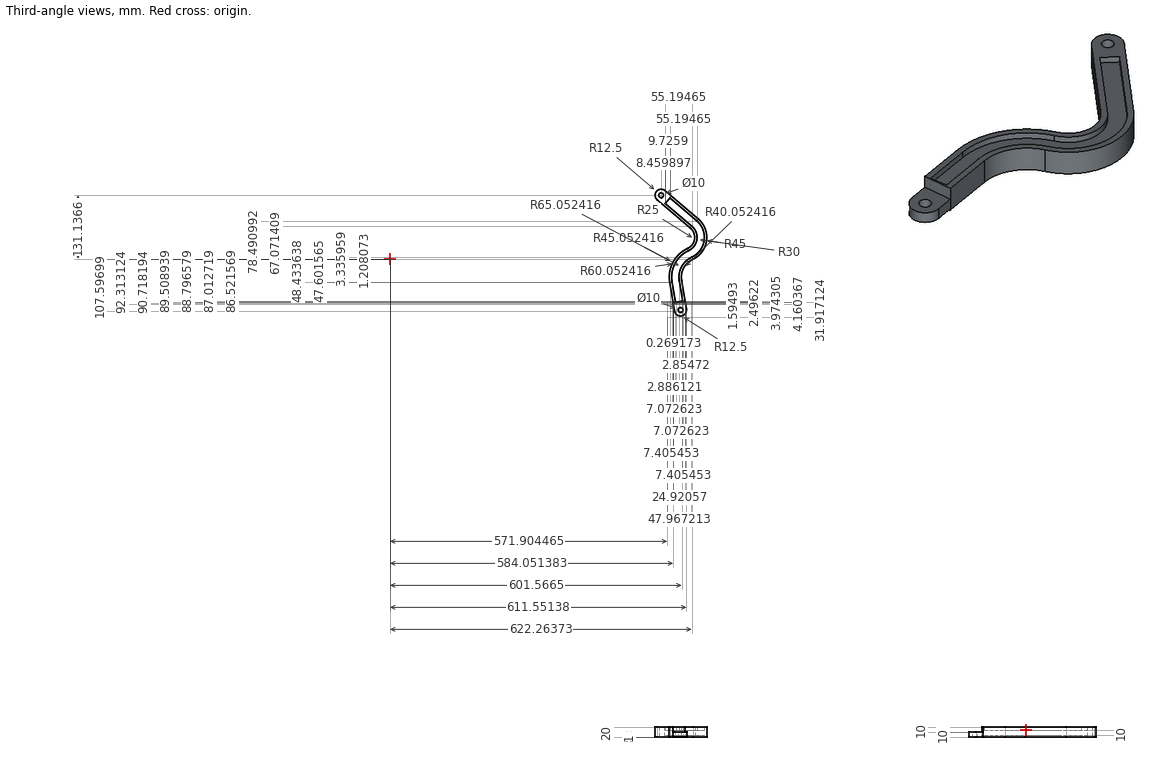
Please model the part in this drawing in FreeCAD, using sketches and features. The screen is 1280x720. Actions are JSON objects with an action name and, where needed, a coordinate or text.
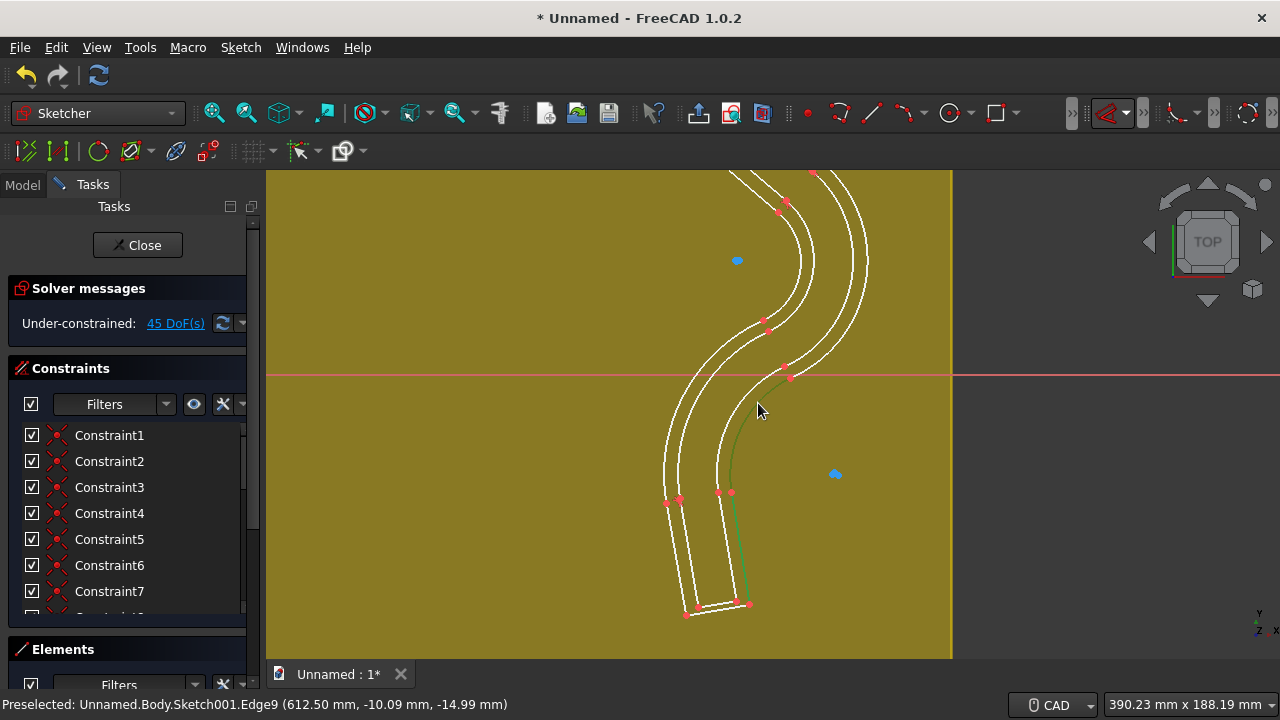
{"action": "key", "text": "t"}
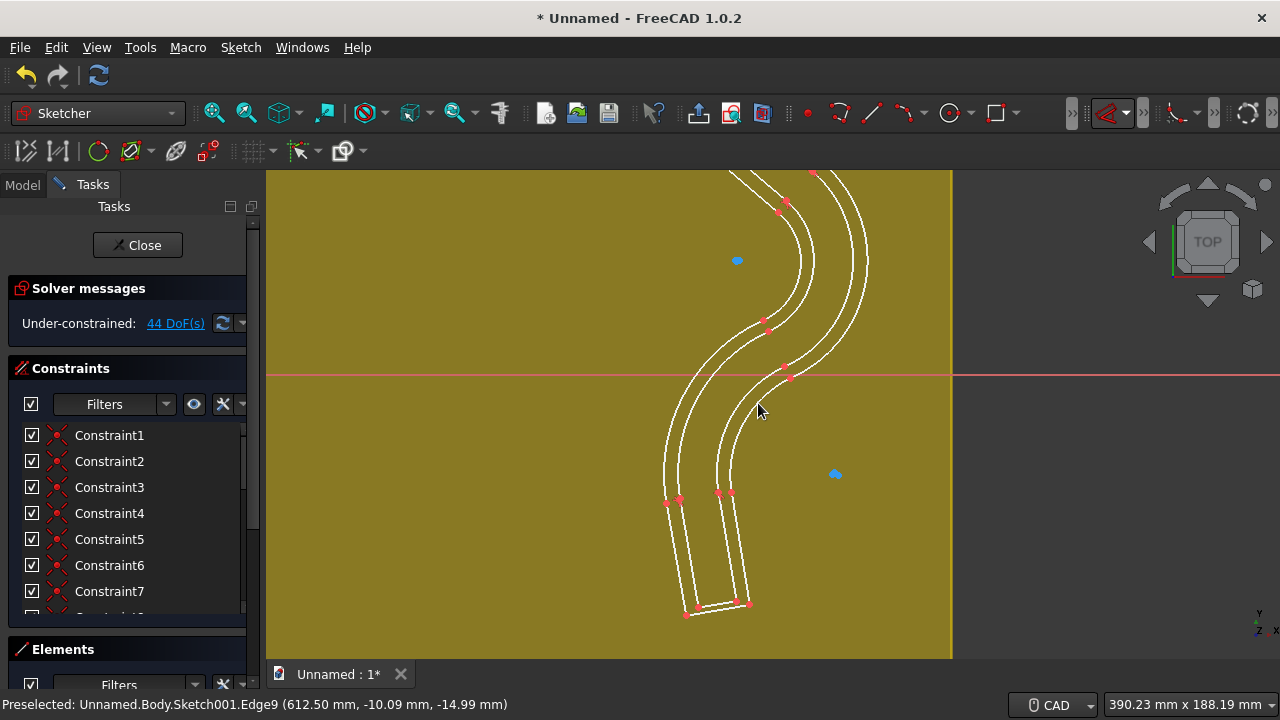
{"action": "left_click", "coordinate": [792, 294]}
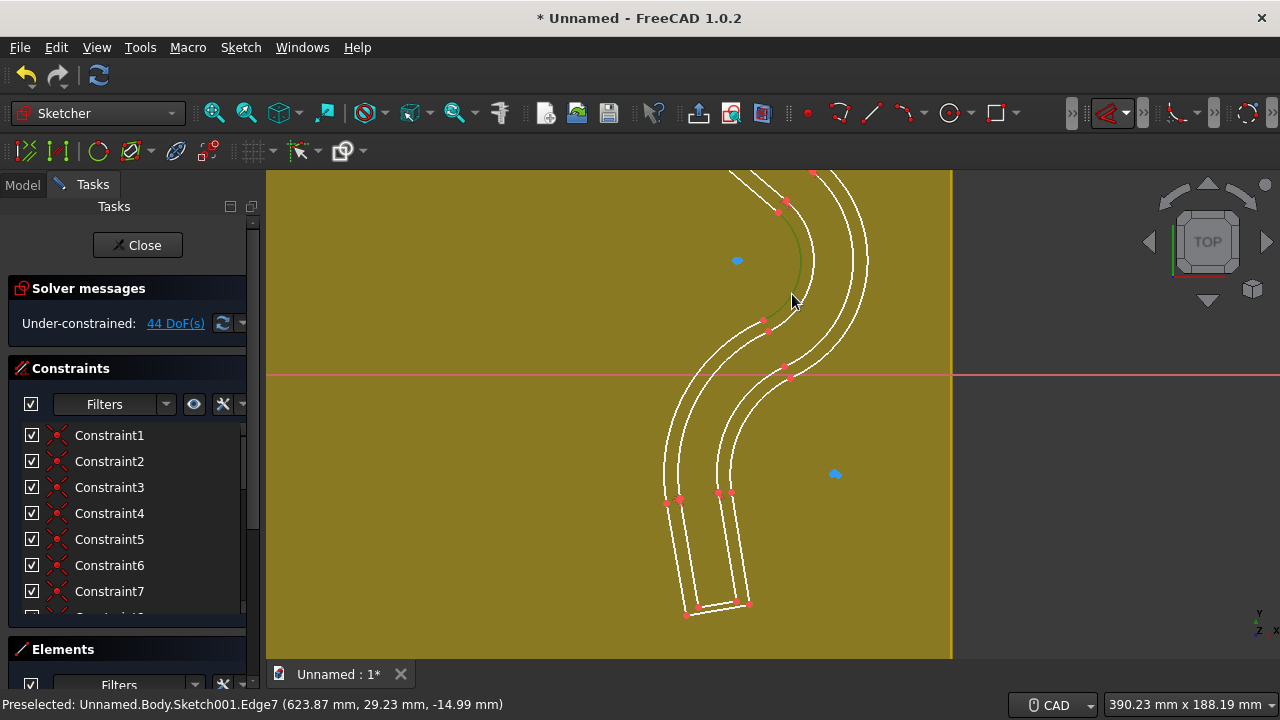
{"action": "left_click", "coordinate": [710, 359]}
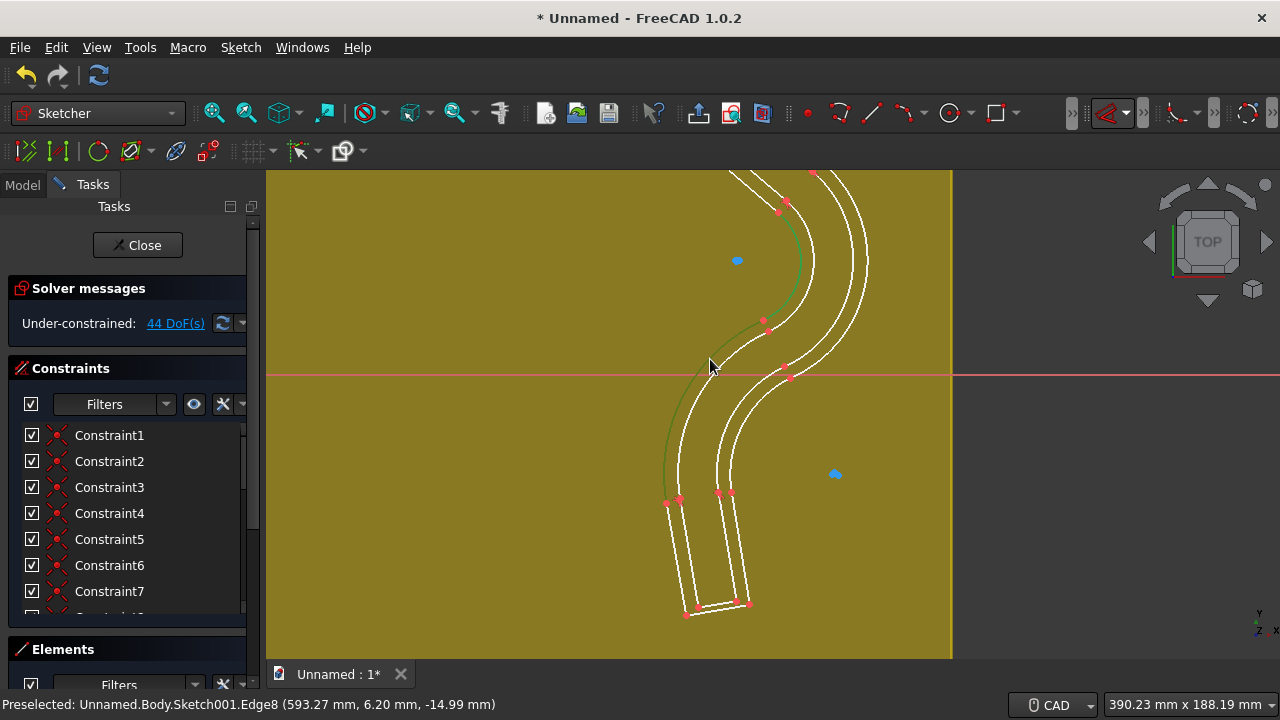
{"action": "key", "text": "t"}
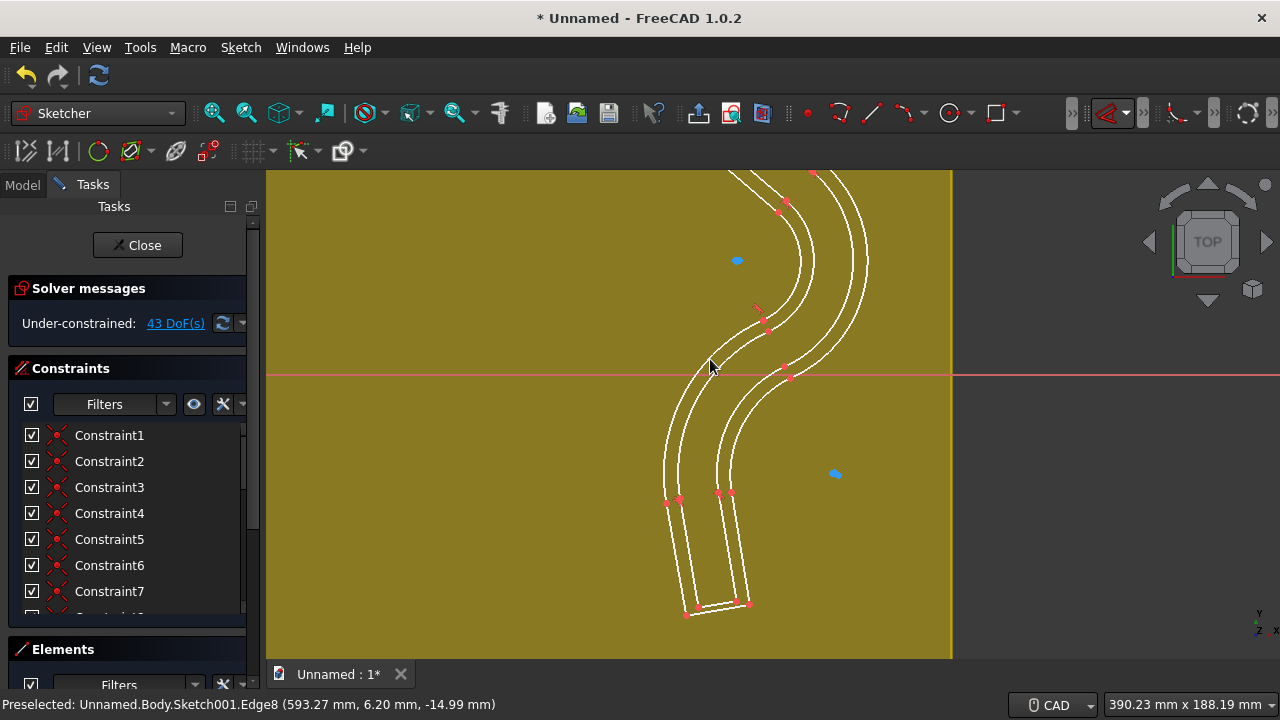
{"action": "left_click", "coordinate": [758, 403]}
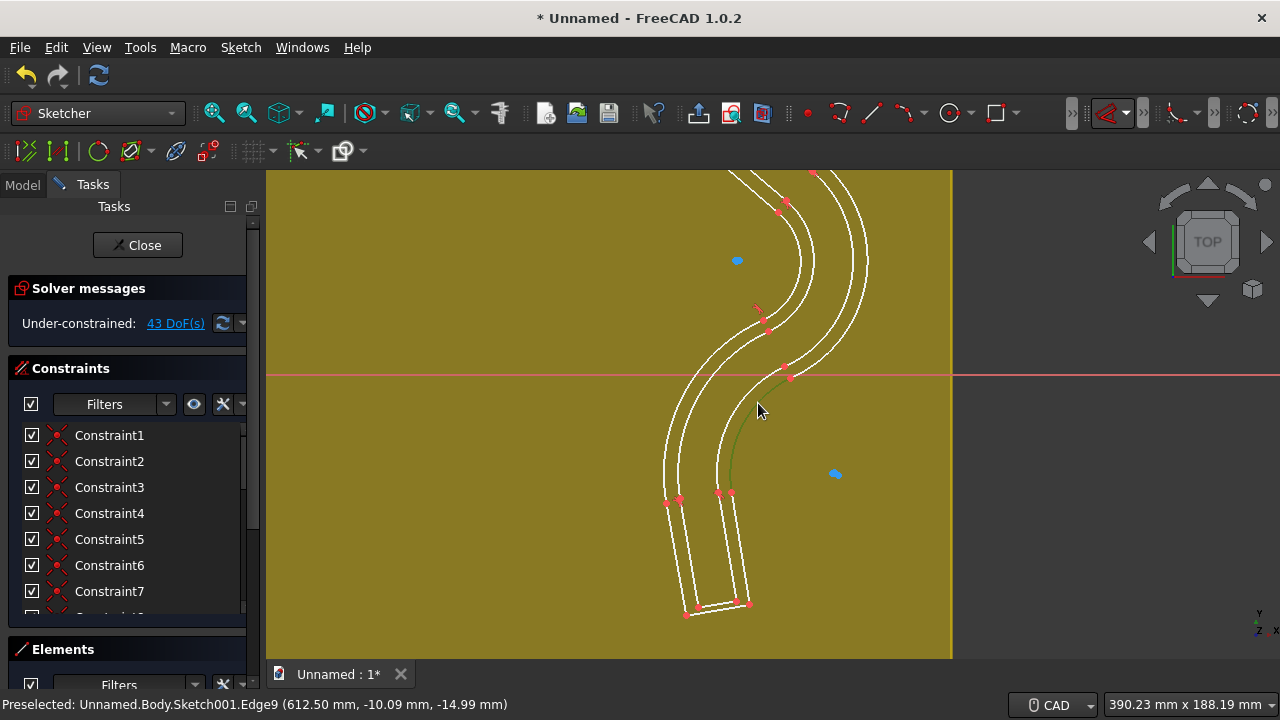
{"action": "left_click", "coordinate": [849, 328]}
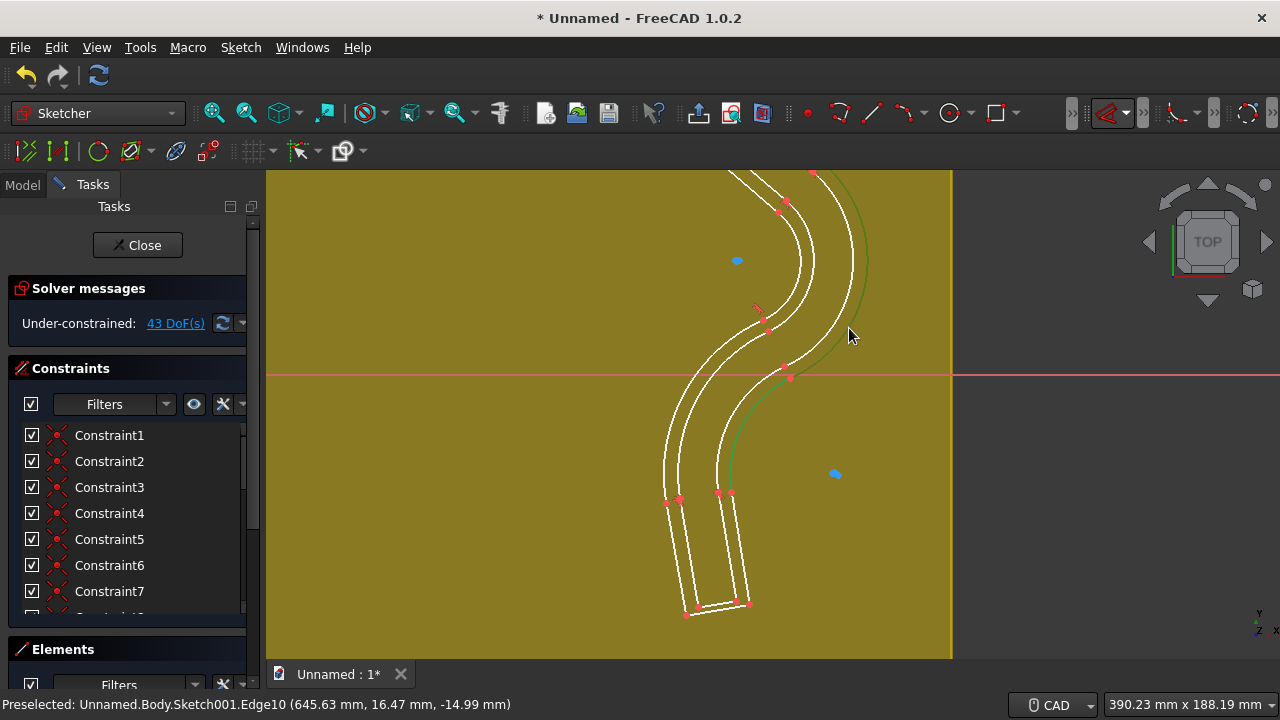
{"action": "key", "text": "t"}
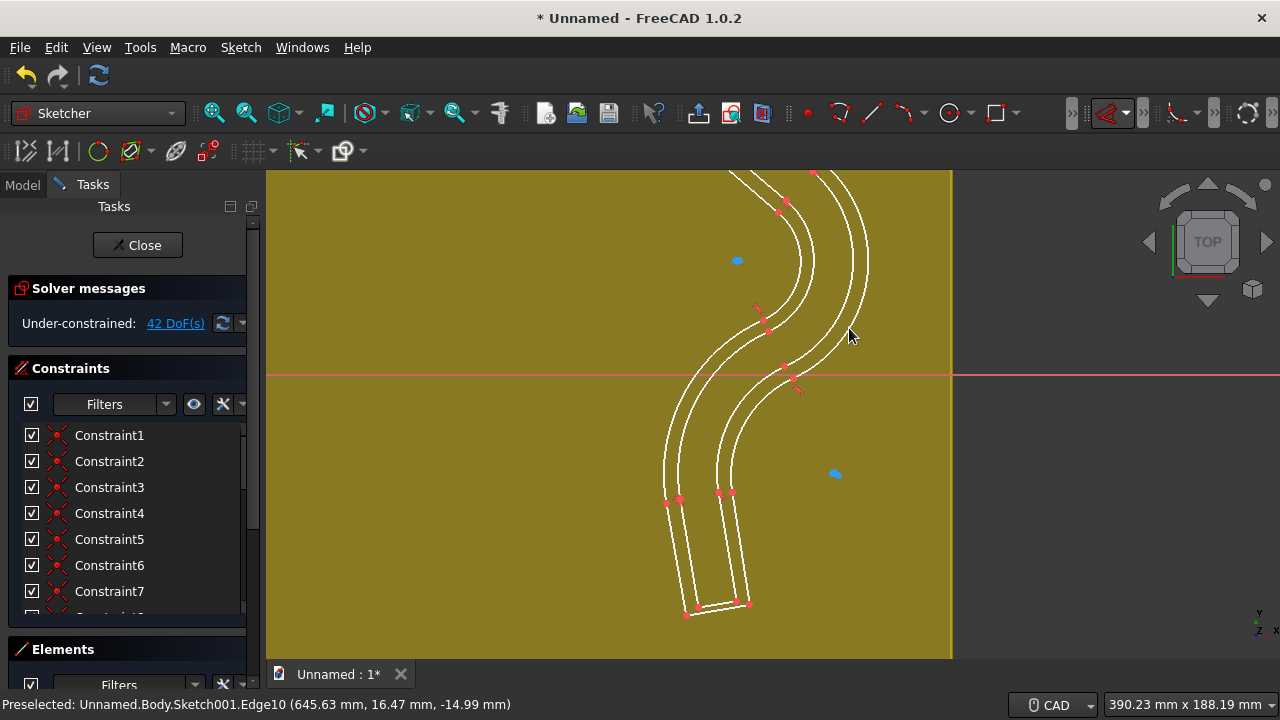
{"action": "left_click", "coordinate": [724, 525]}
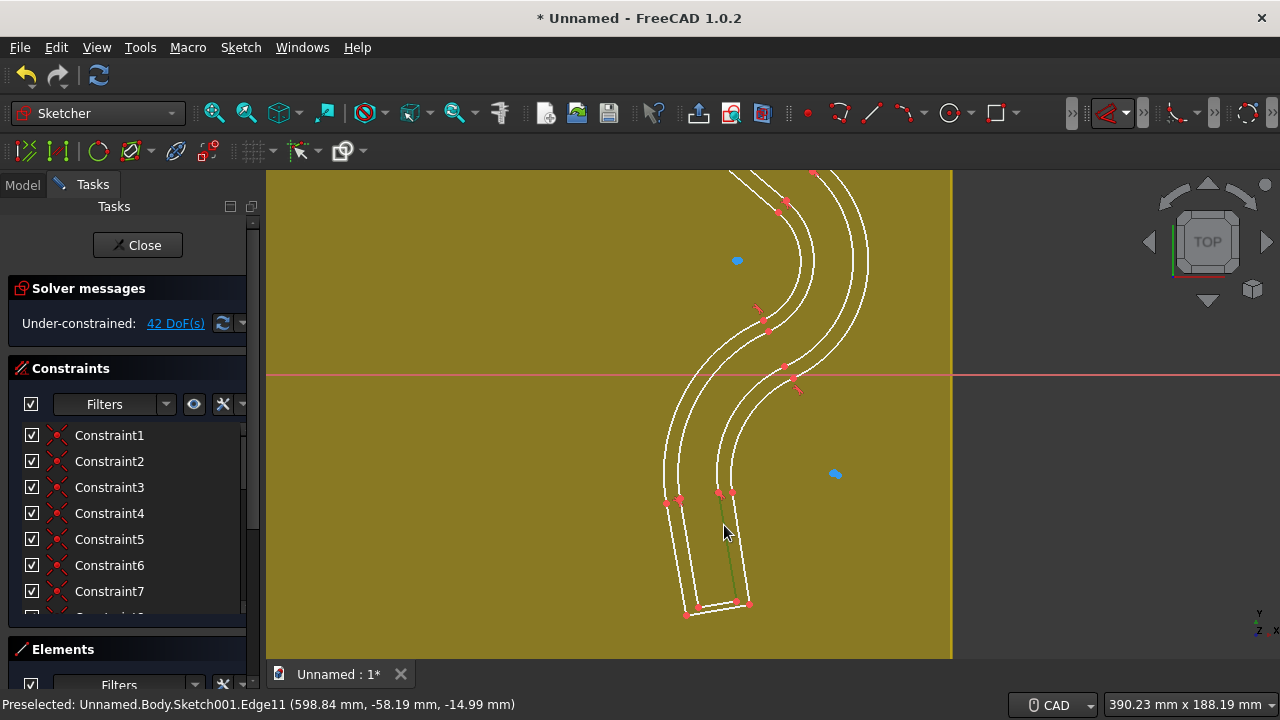
{"action": "left_click", "coordinate": [748, 393]}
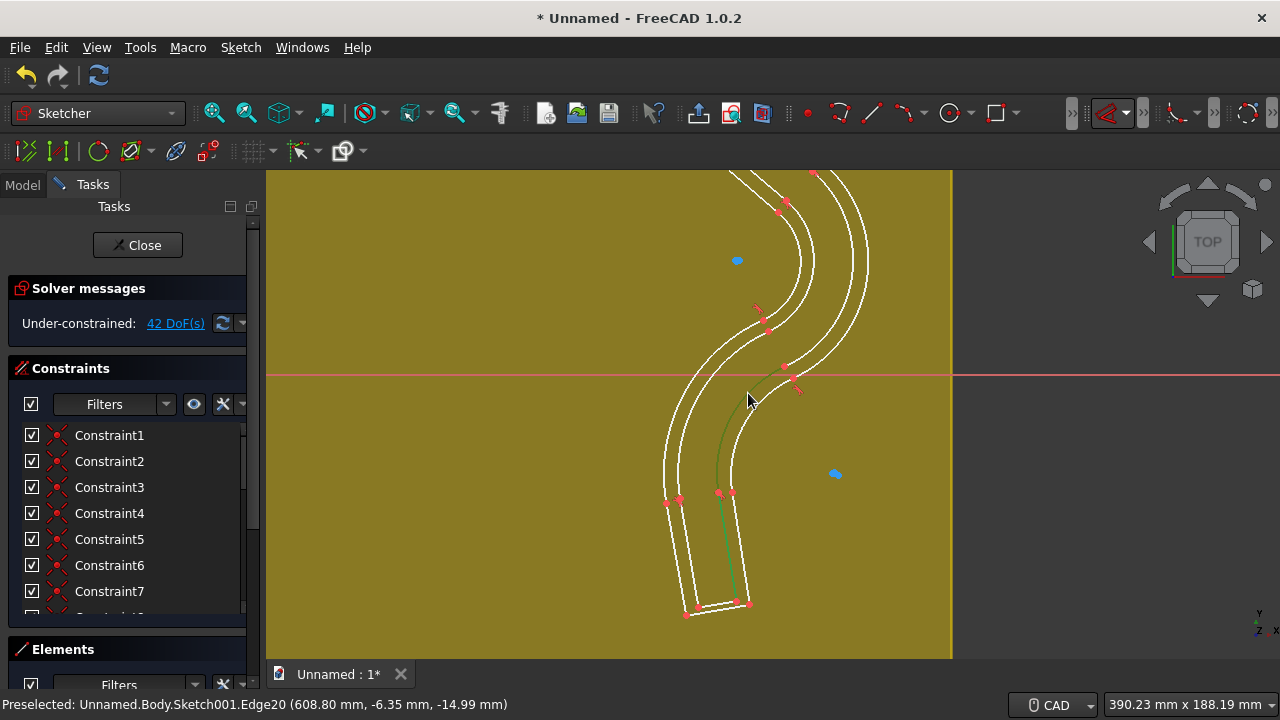
{"action": "key", "text": "t"}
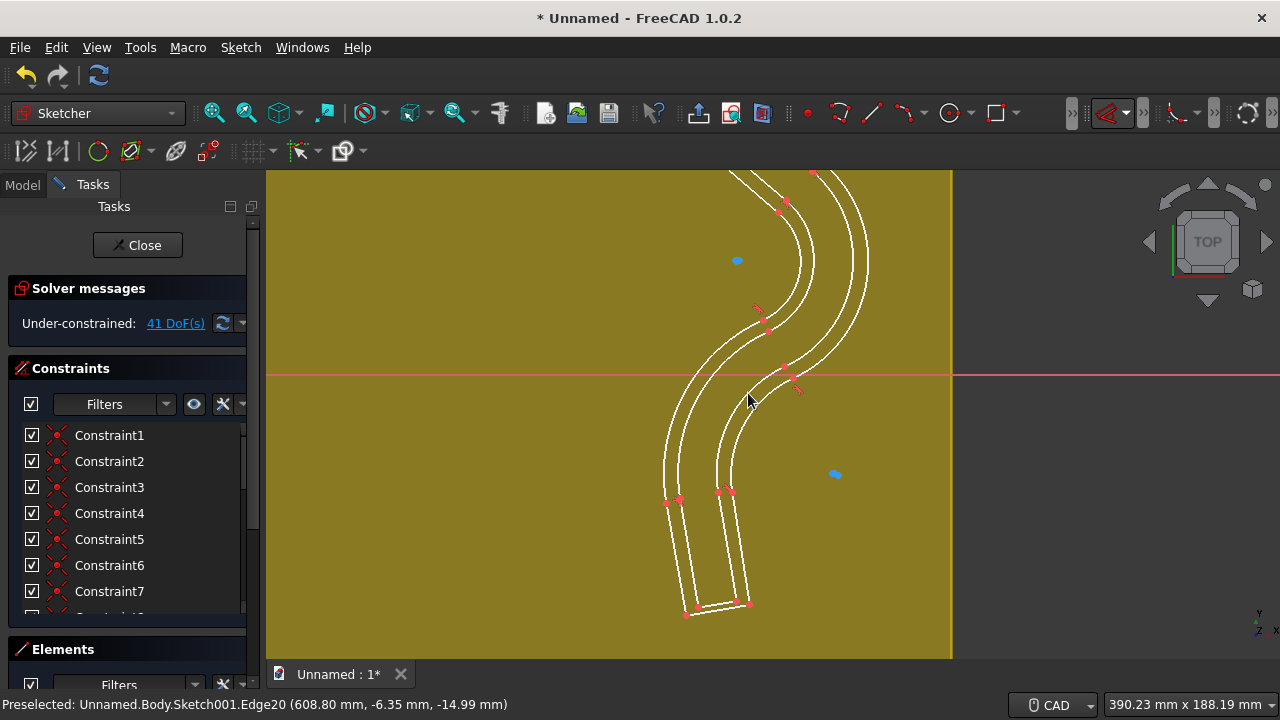
{"action": "left_click", "coordinate": [693, 575]}